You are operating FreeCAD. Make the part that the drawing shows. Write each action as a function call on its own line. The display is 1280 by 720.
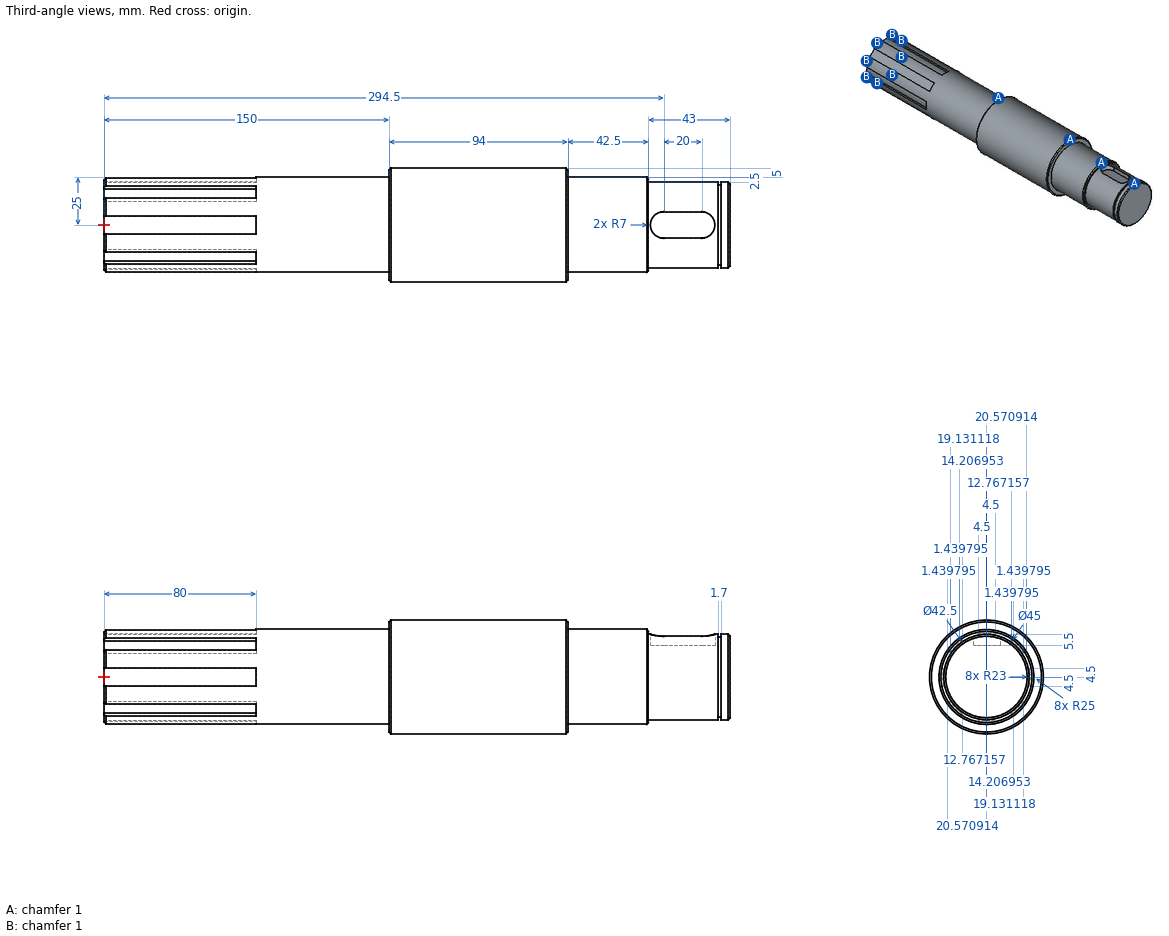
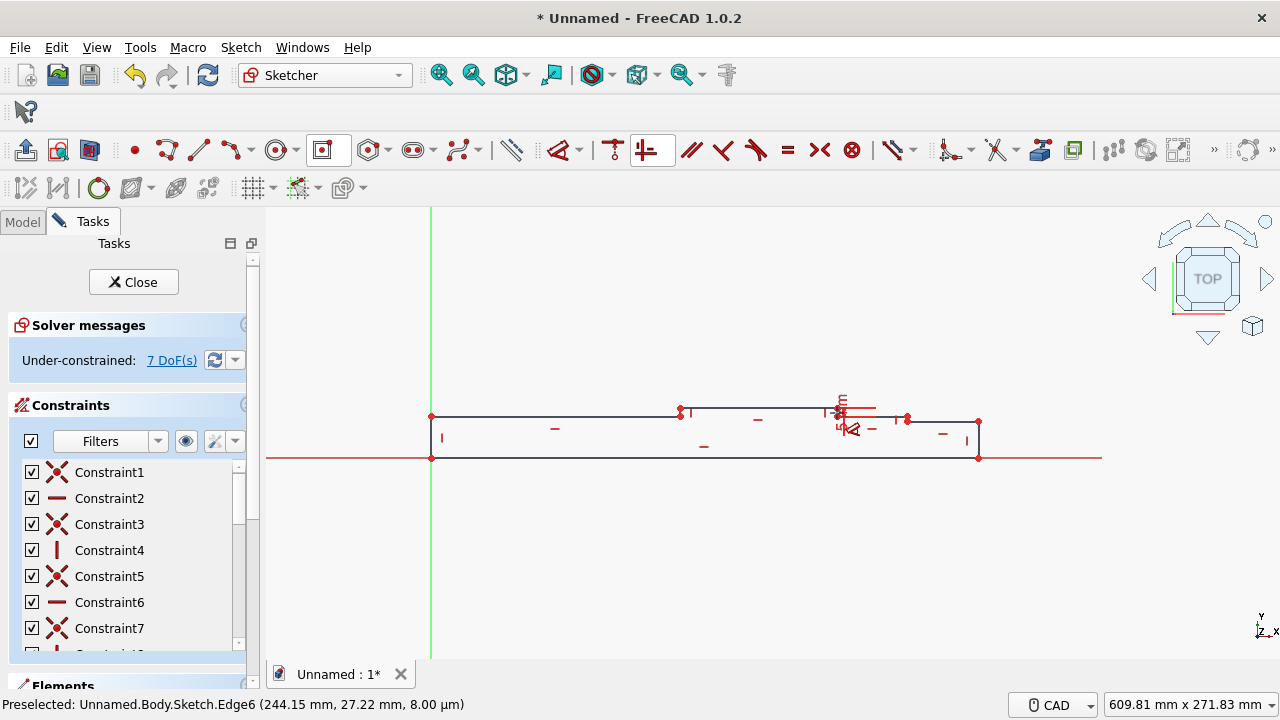
scroll(680, 411, up, 9)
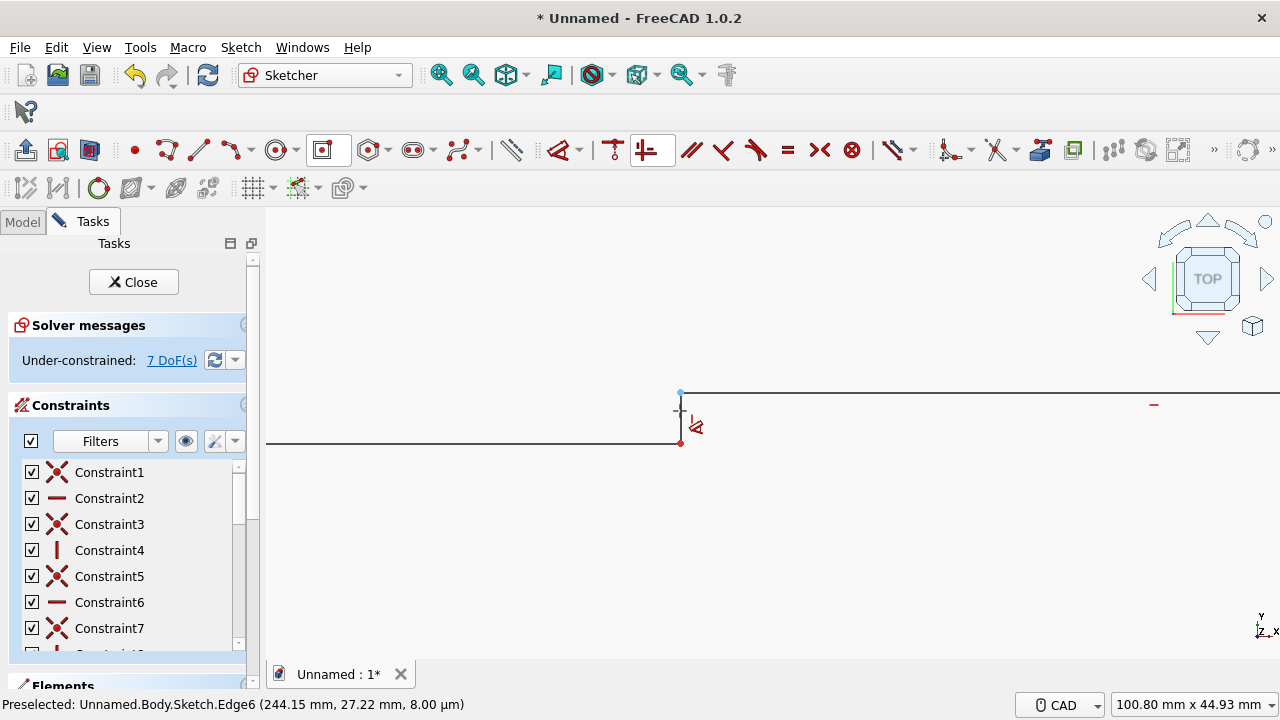
click(681, 408)
click(647, 418)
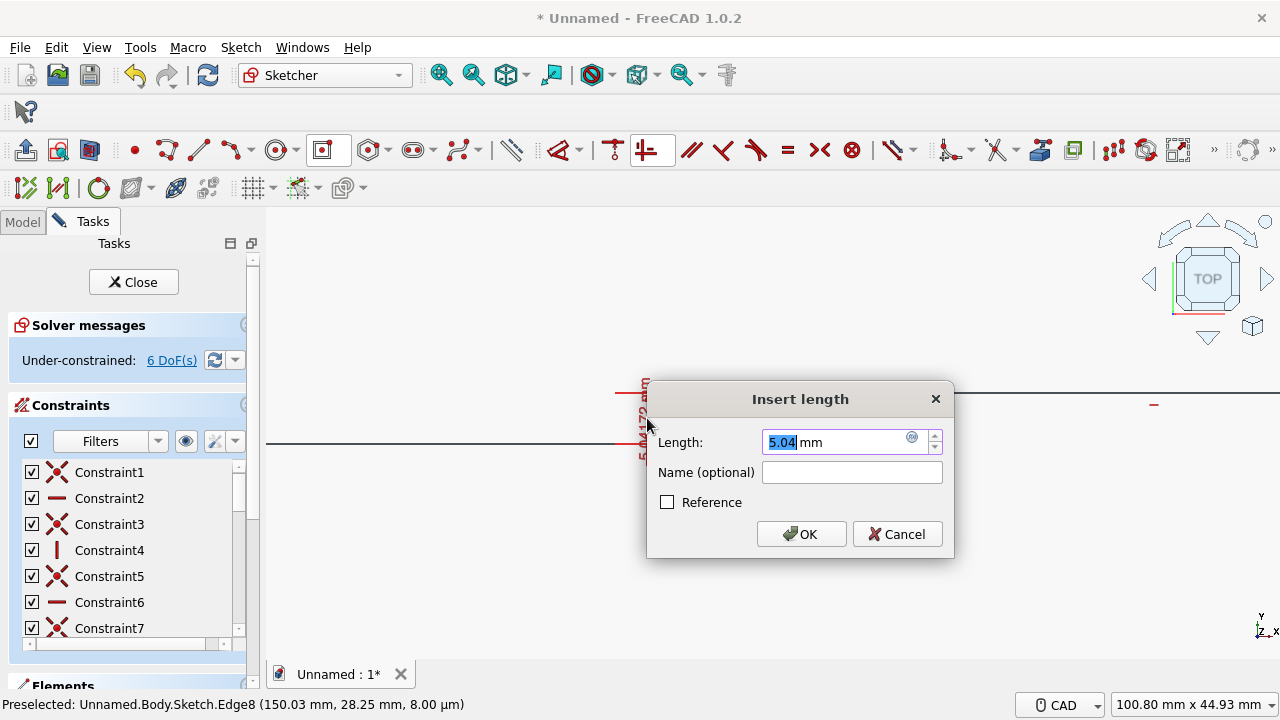
text(5)
key(Return)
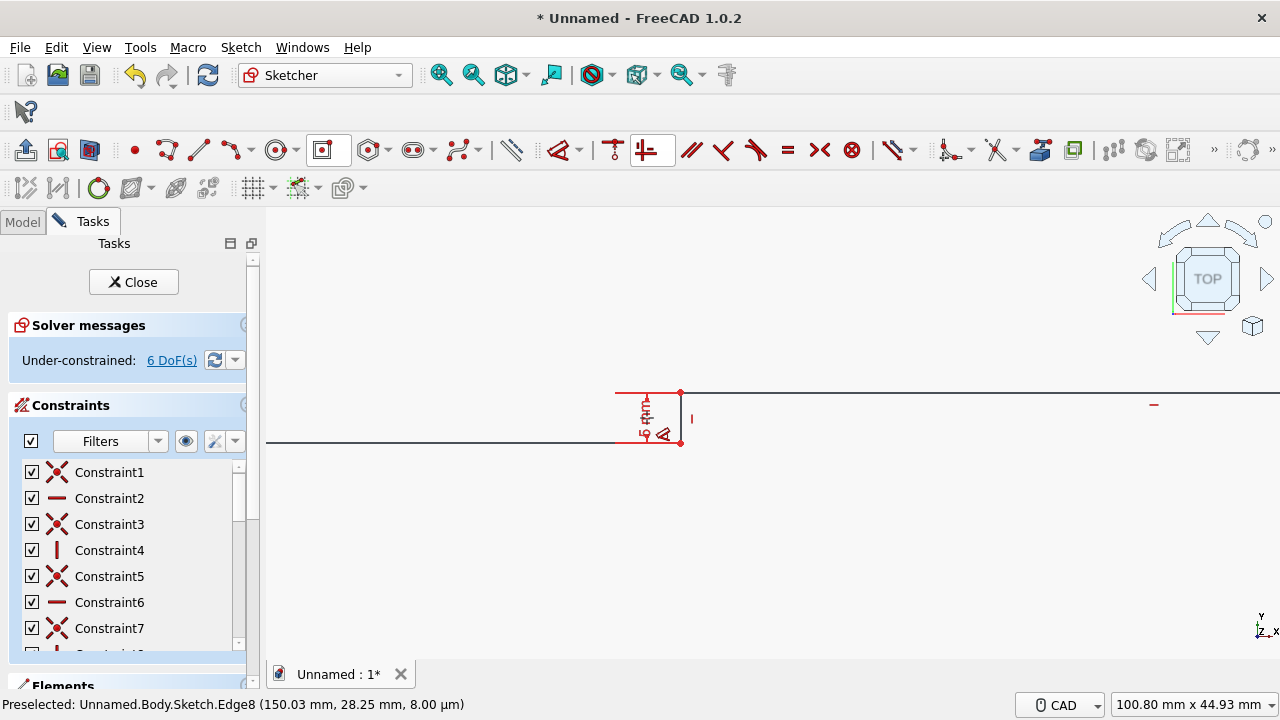
scroll(680, 411, down, 9)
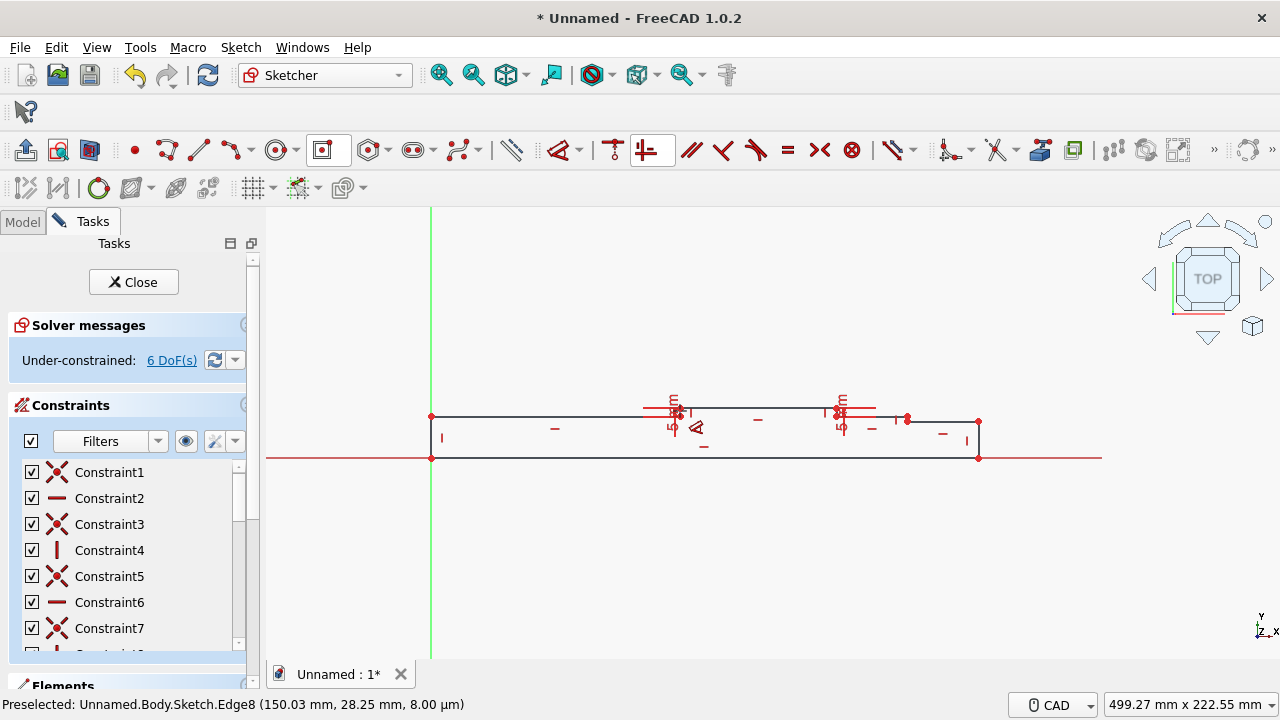
click(957, 422)
click(943, 388)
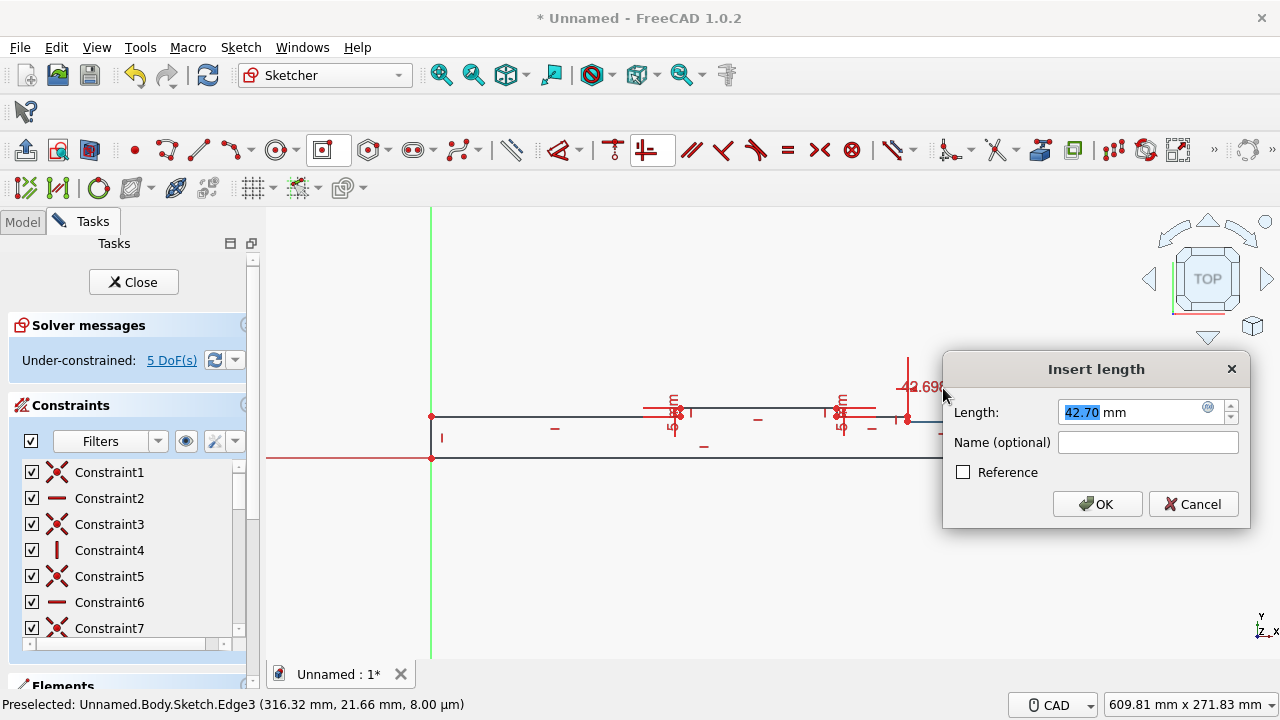
text(43)
key(Return)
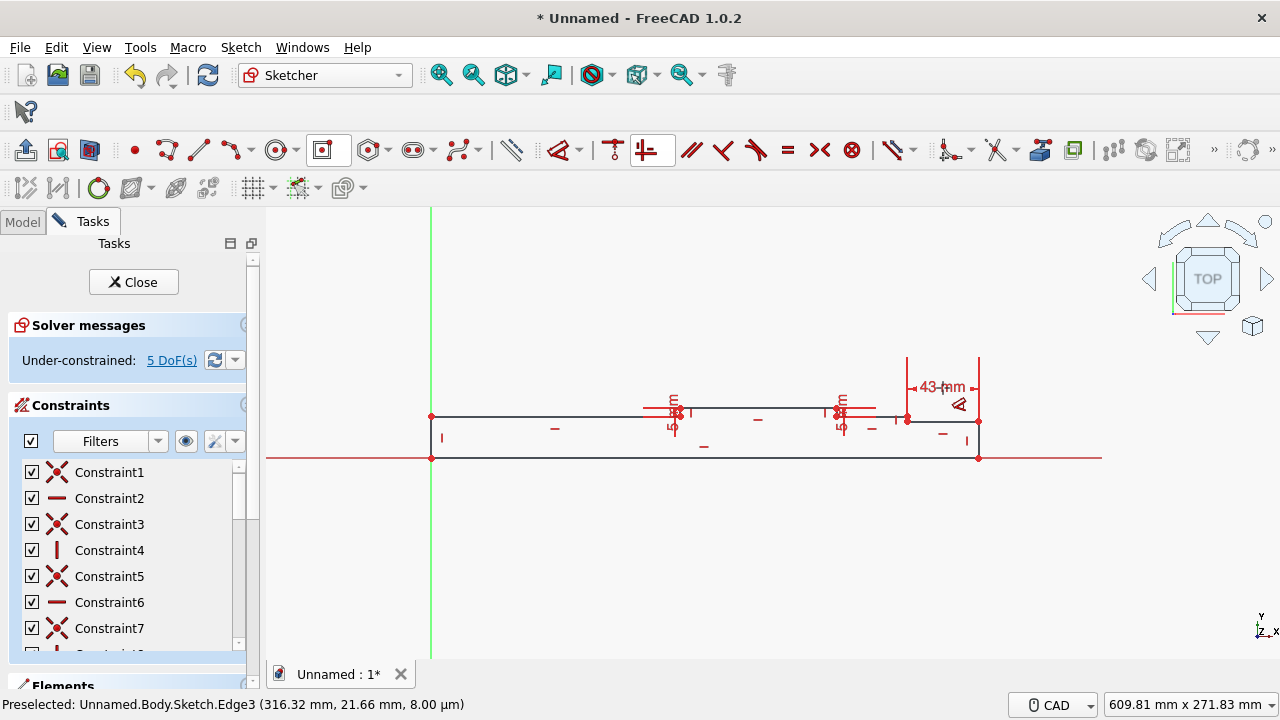
click(790, 408)
click(759, 374)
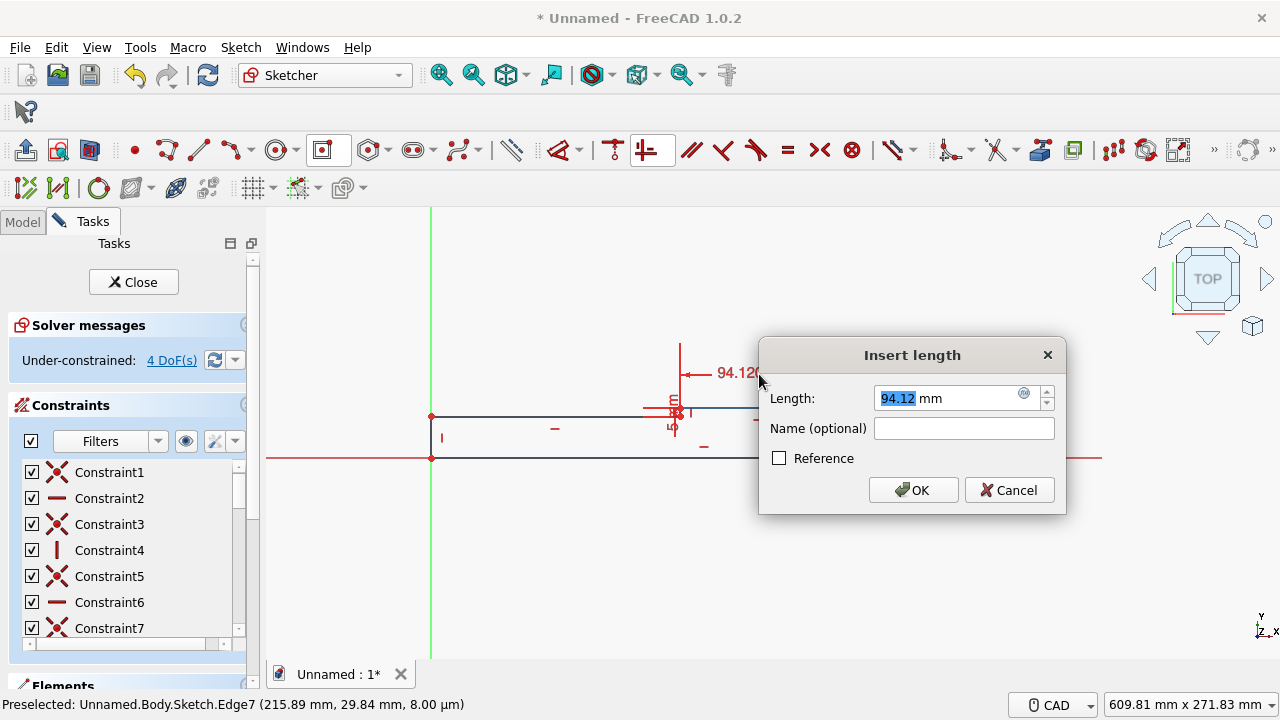
text(94)
key(Return)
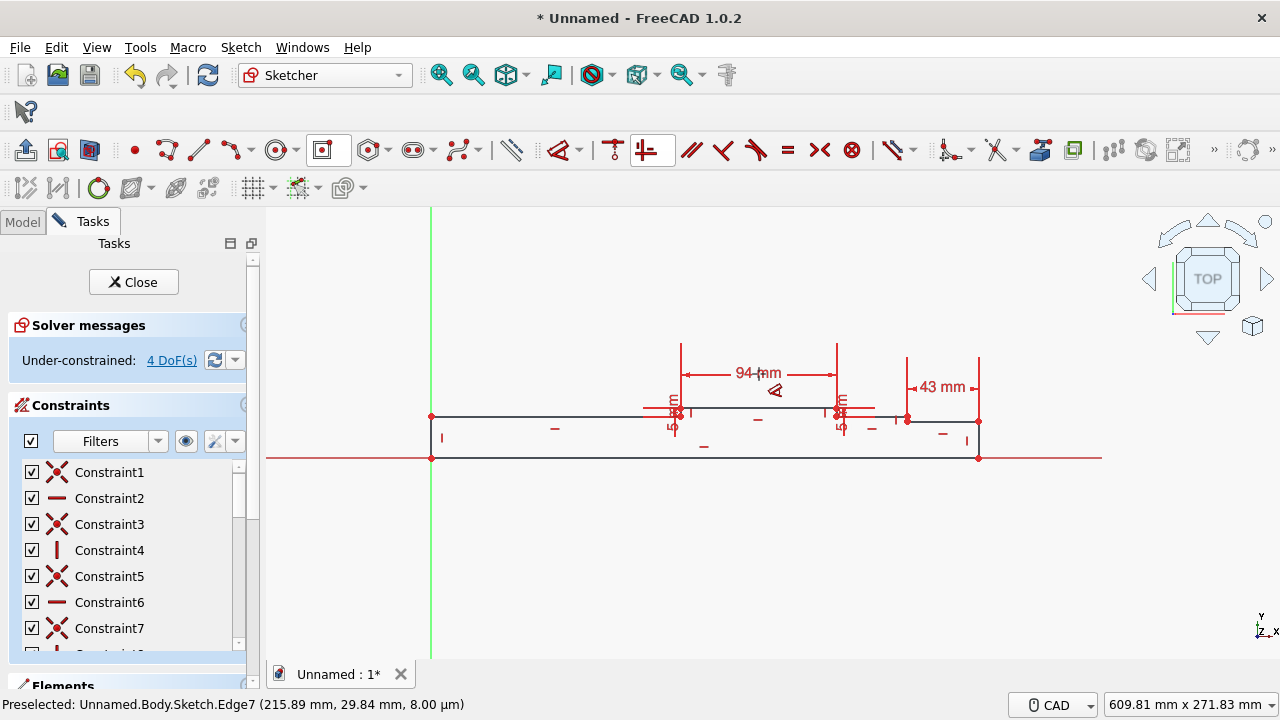
click(431, 429)
click(397, 437)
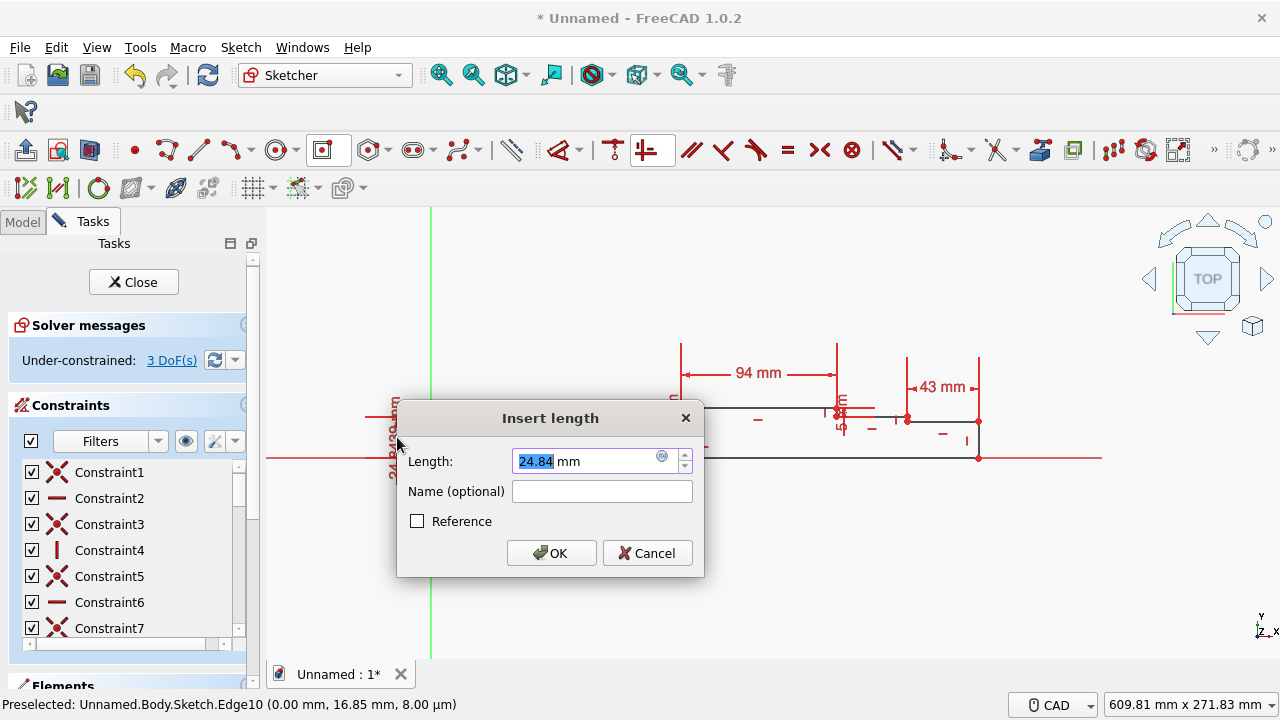
text(25)
key(Return)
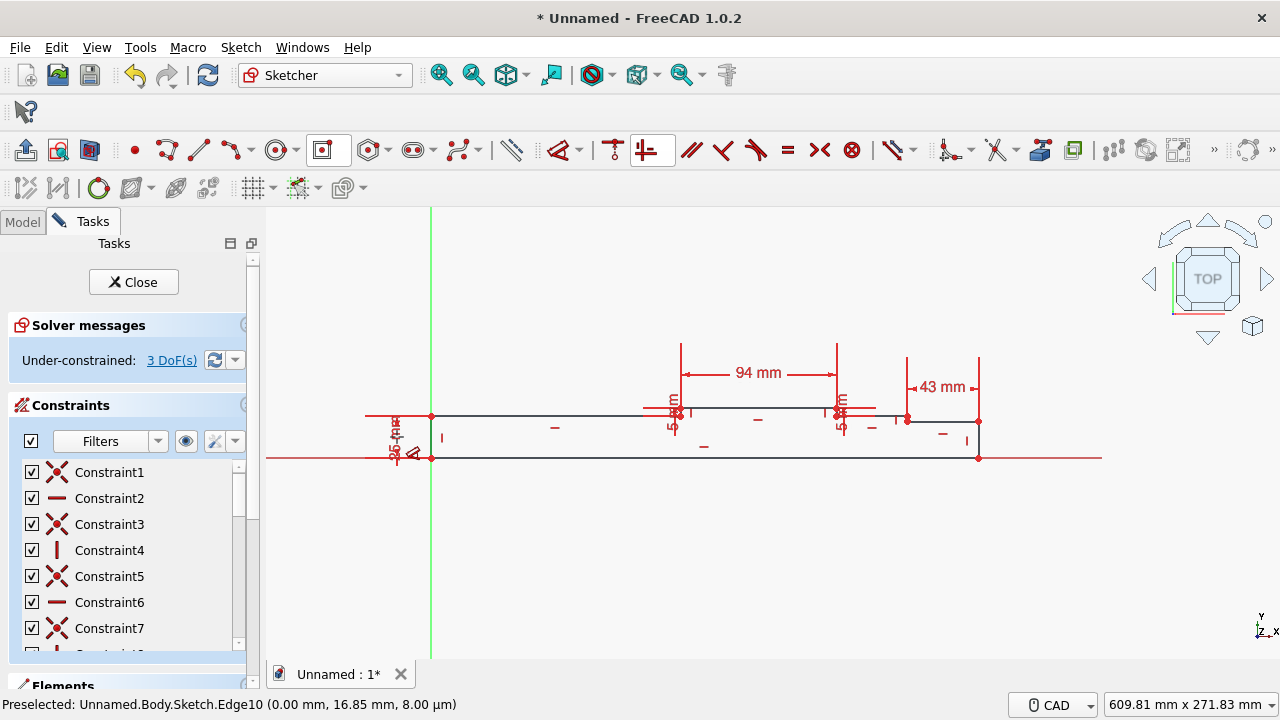
scroll(907, 419, up, 12)